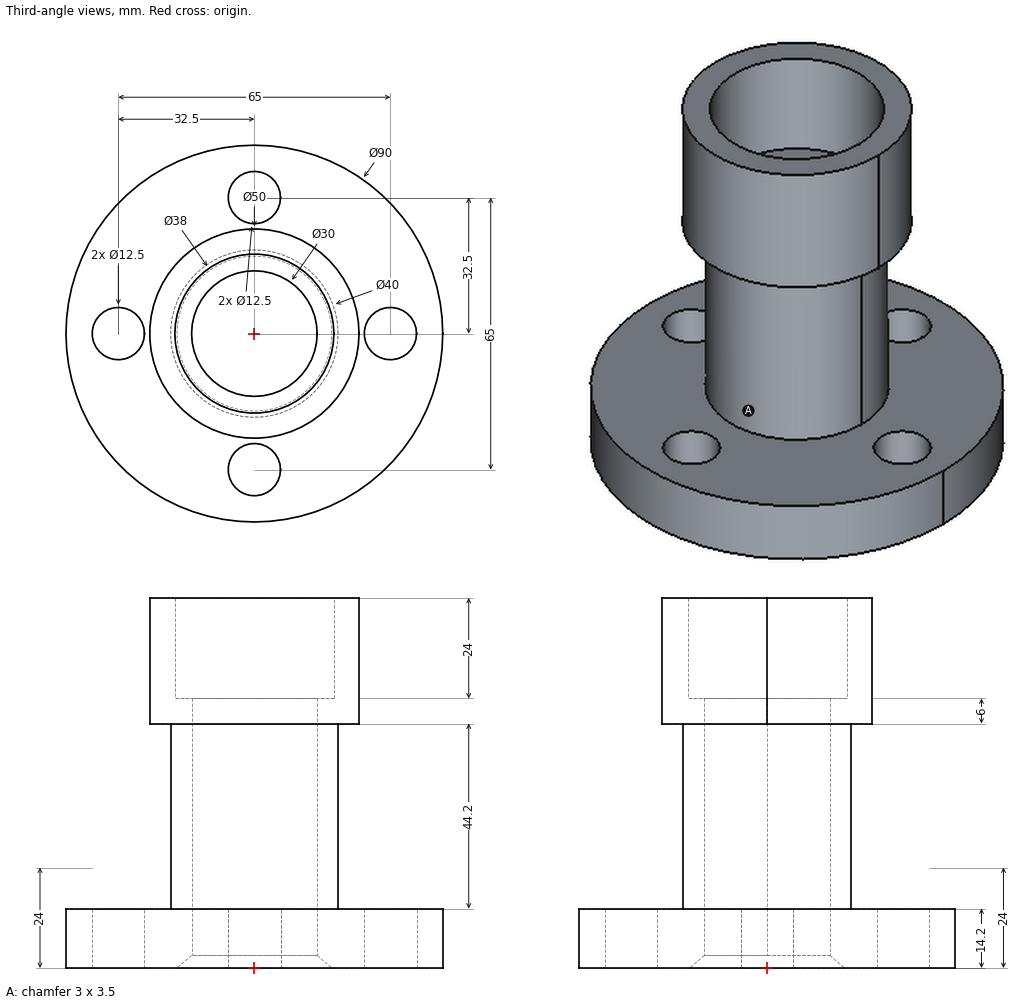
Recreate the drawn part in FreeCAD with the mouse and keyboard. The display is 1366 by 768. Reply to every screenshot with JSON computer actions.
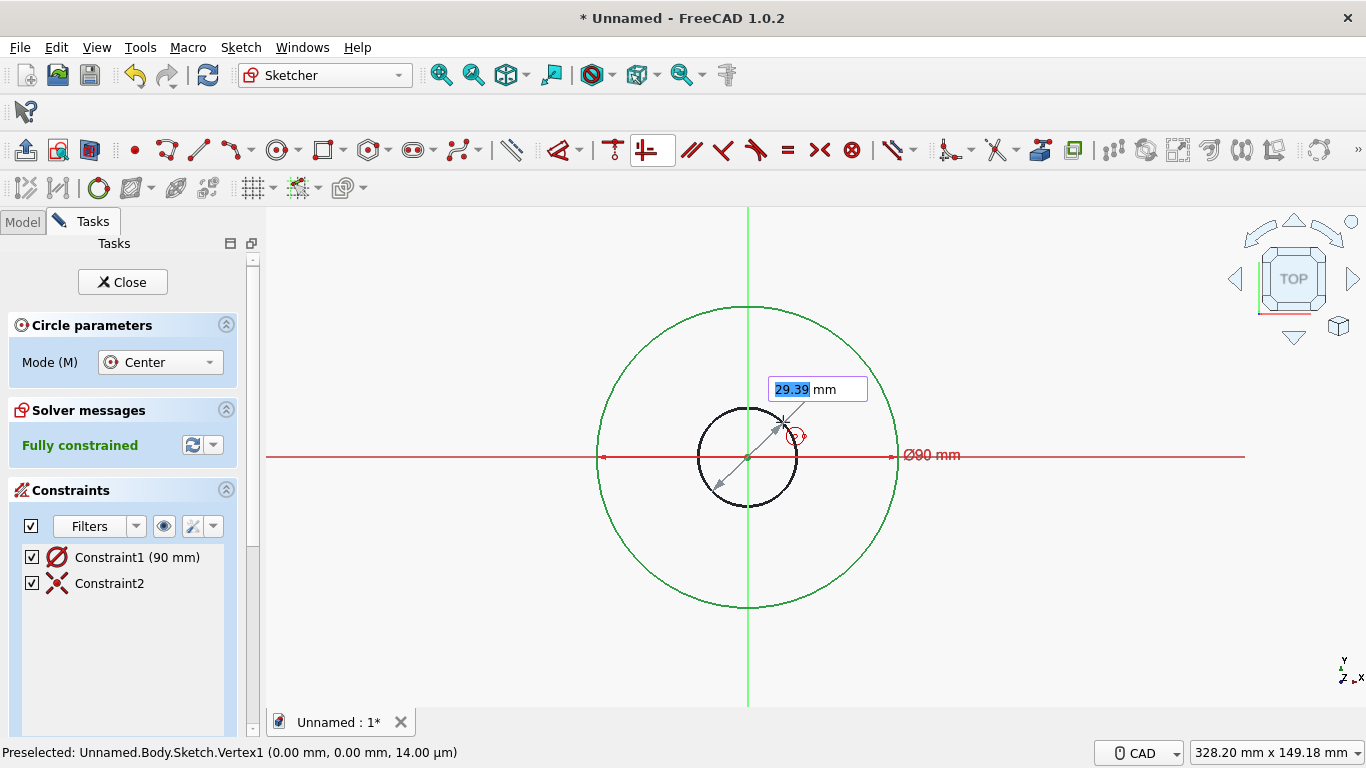
{"action": "type", "text": "30"}
{"action": "key", "text": "Return"}
{"action": "key", "text": "Escape"}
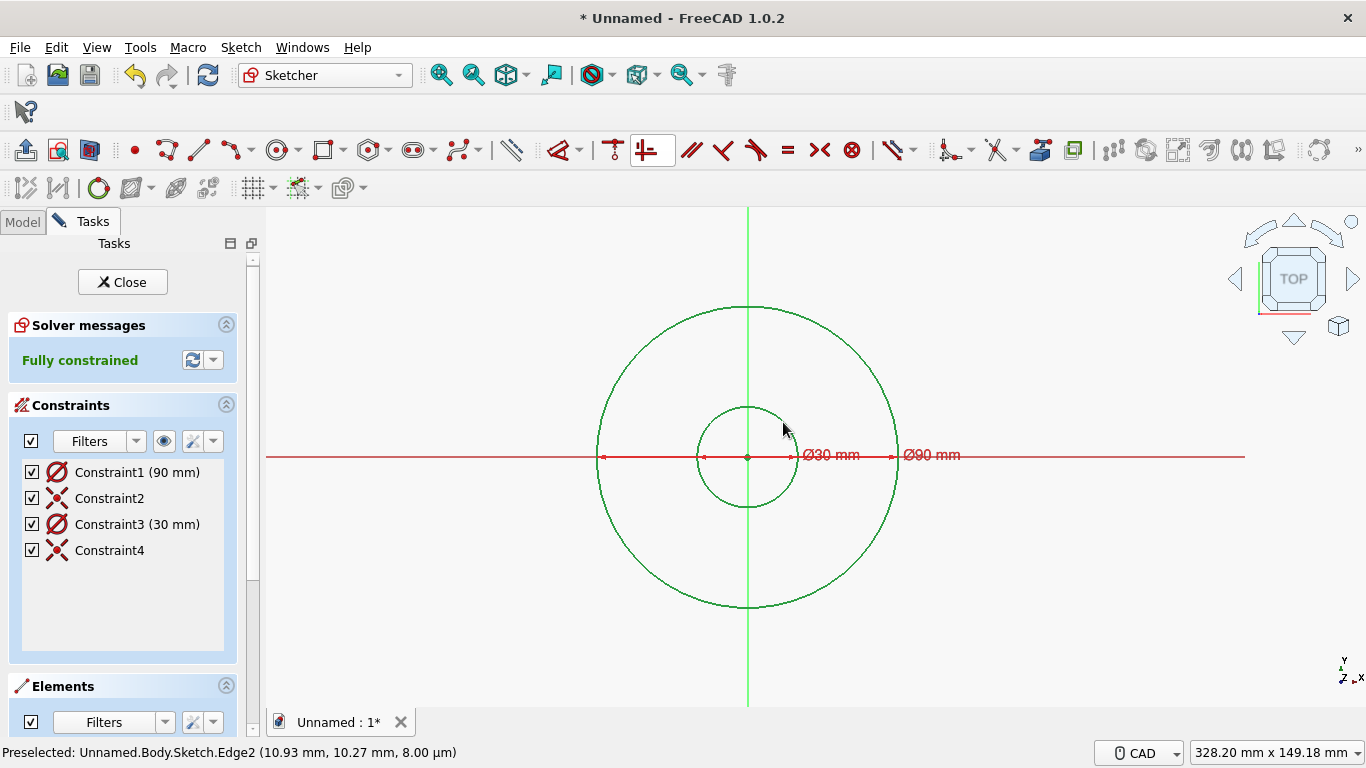
{"action": "left_click", "coordinate": [123, 282]}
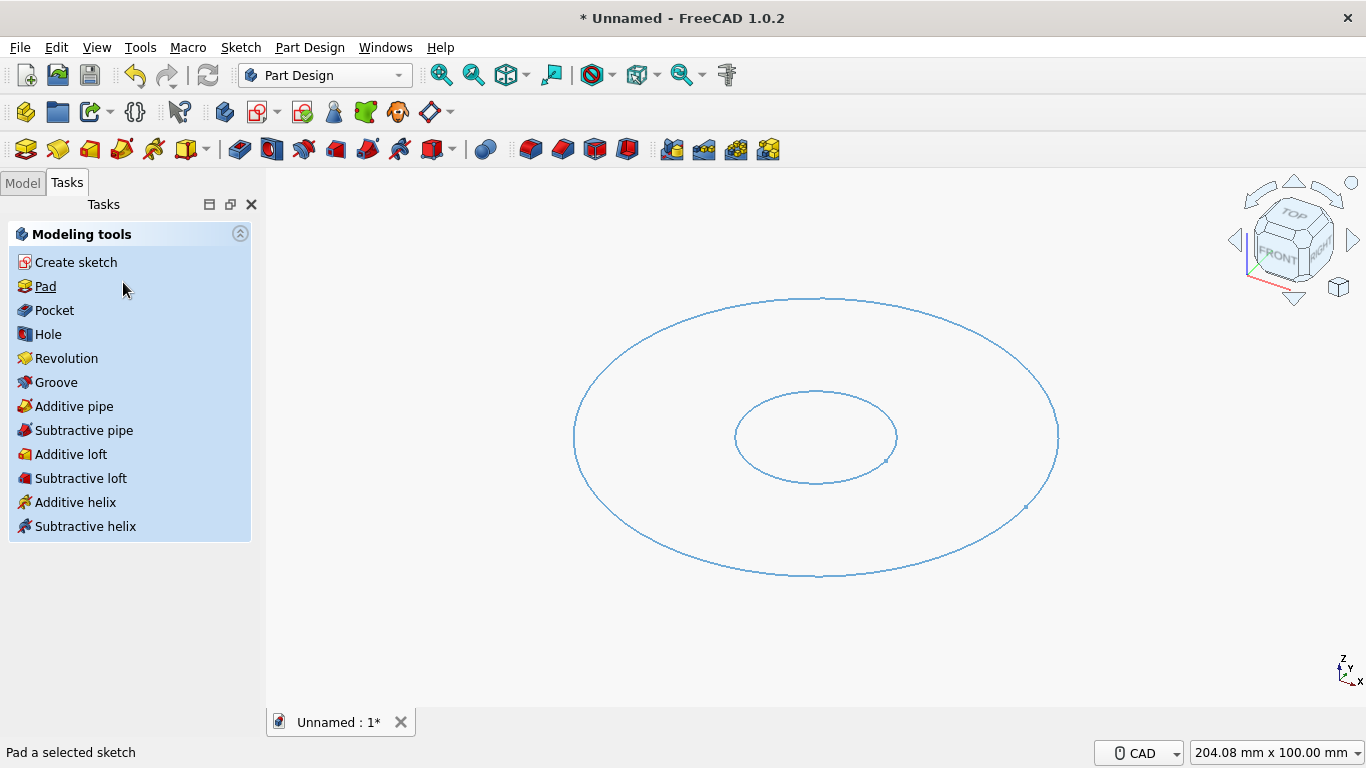
{"action": "left_click", "coordinate": [26, 150]}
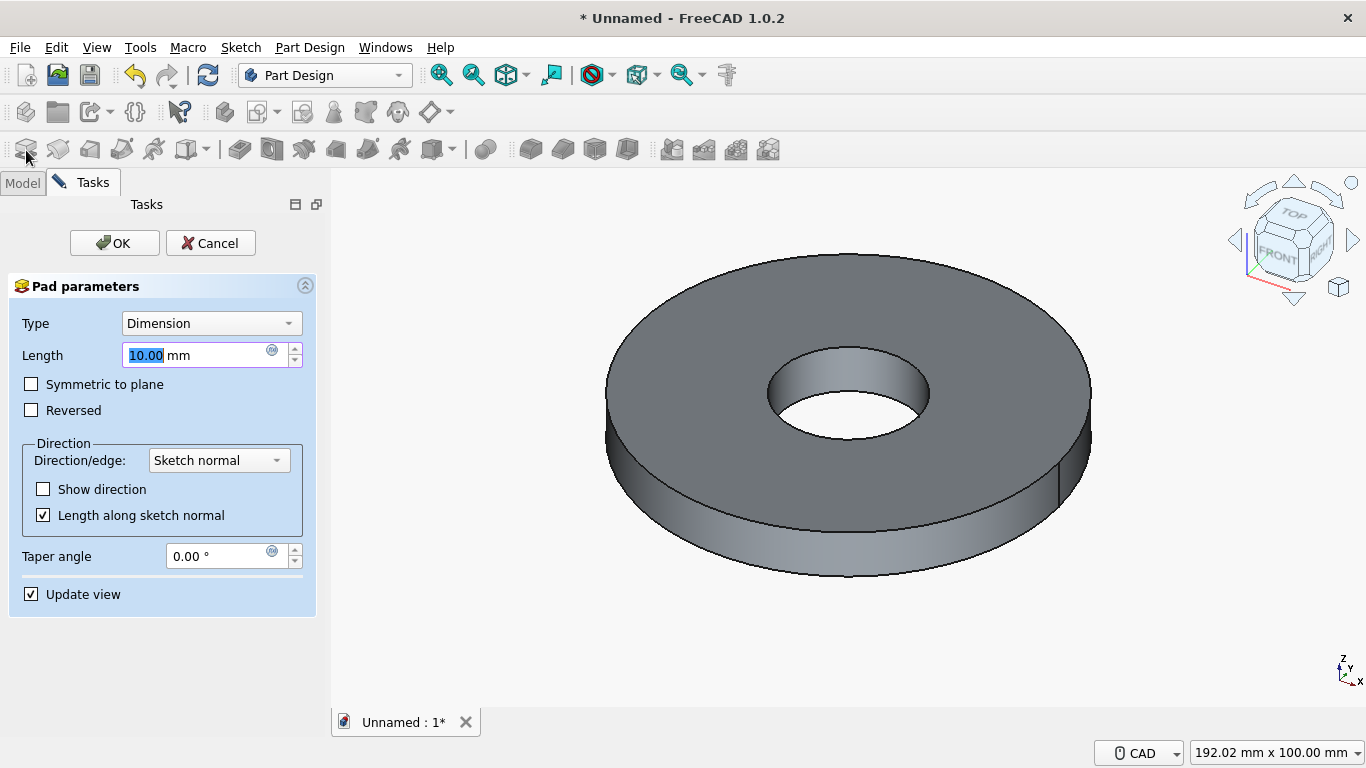
{"action": "type", "text": "14.2"}
{"action": "key", "text": "Tab"}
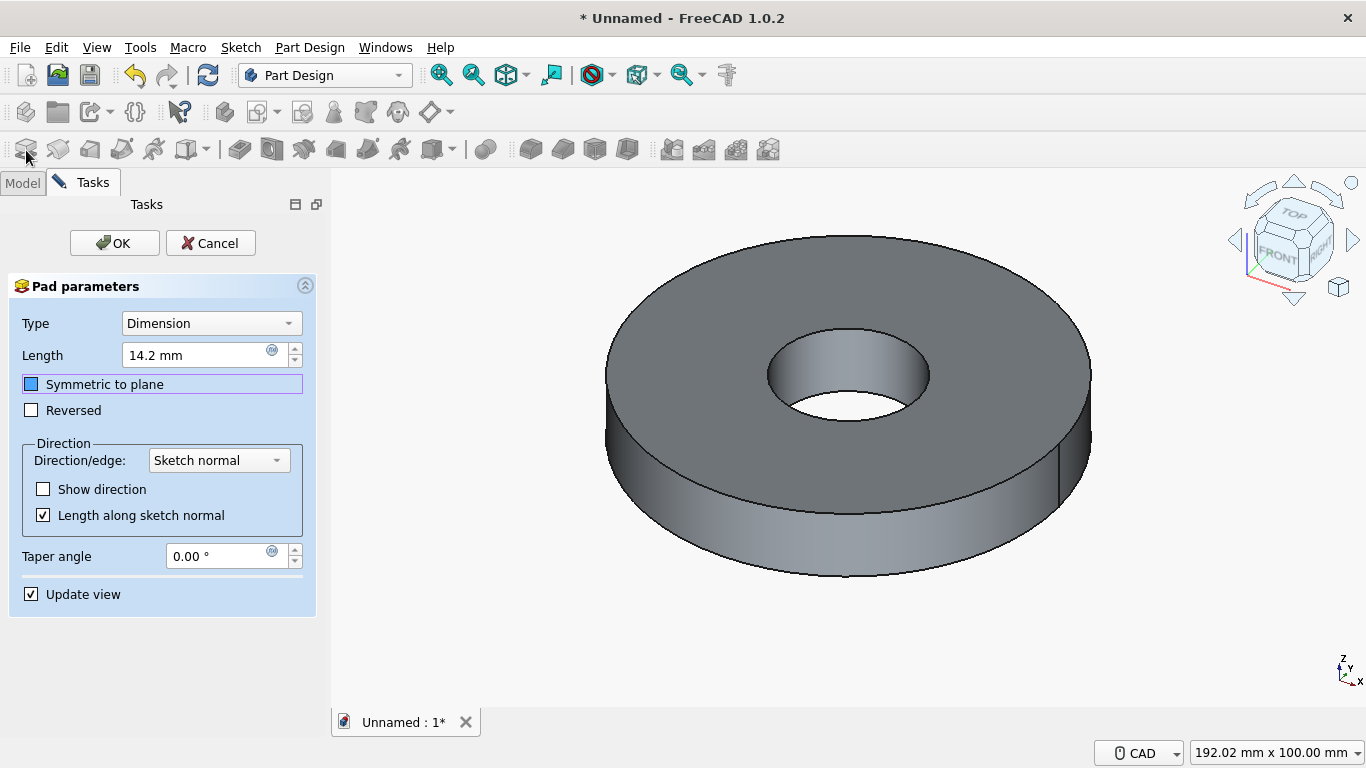
{"action": "left_click", "coordinate": [115, 243]}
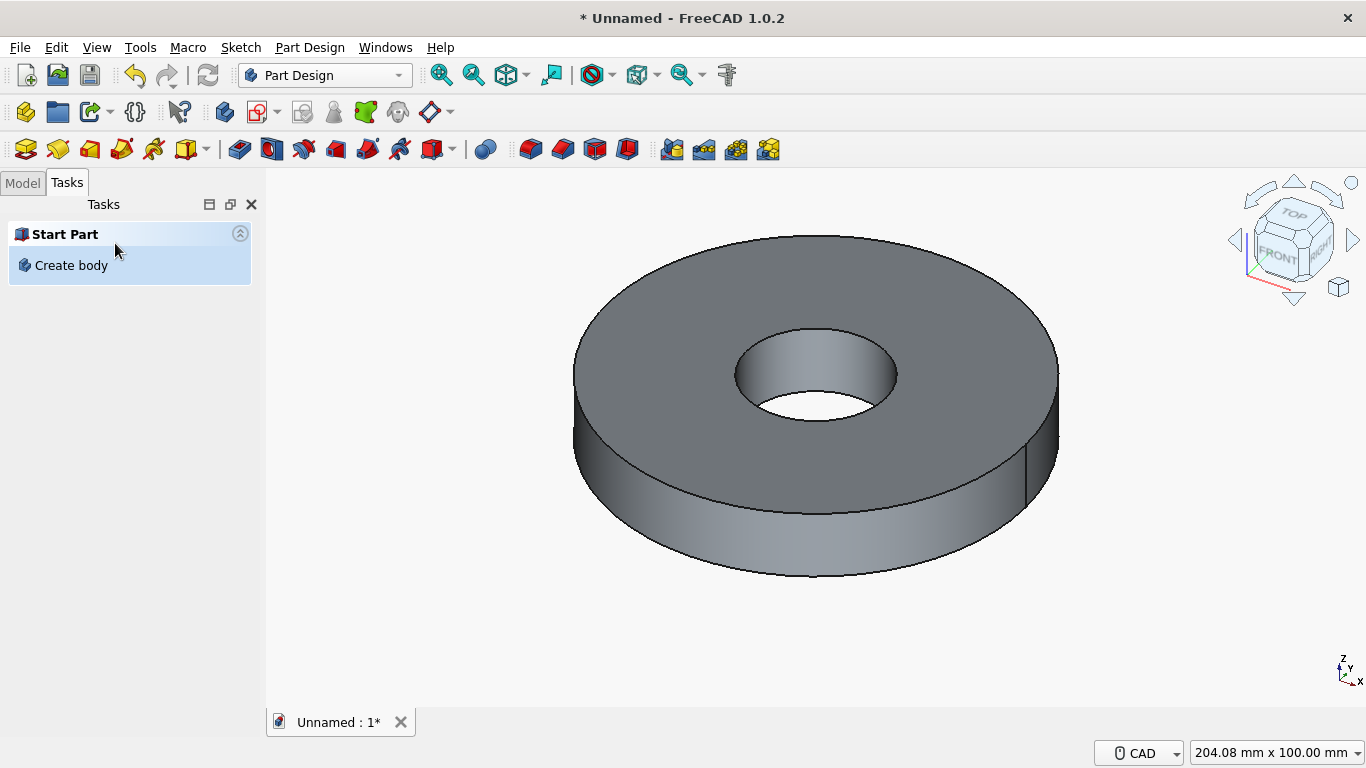
{"action": "left_click", "coordinate": [687, 423]}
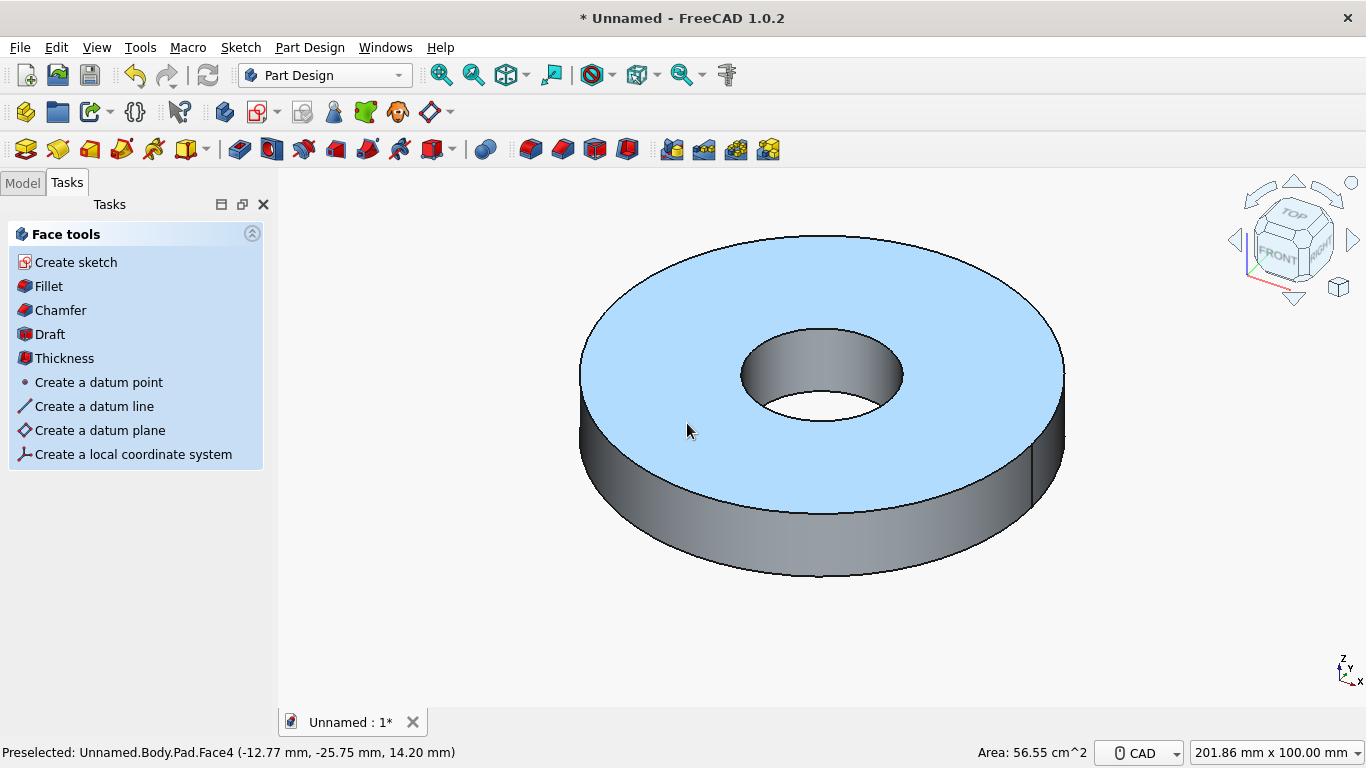
{"action": "left_click", "coordinate": [258, 112]}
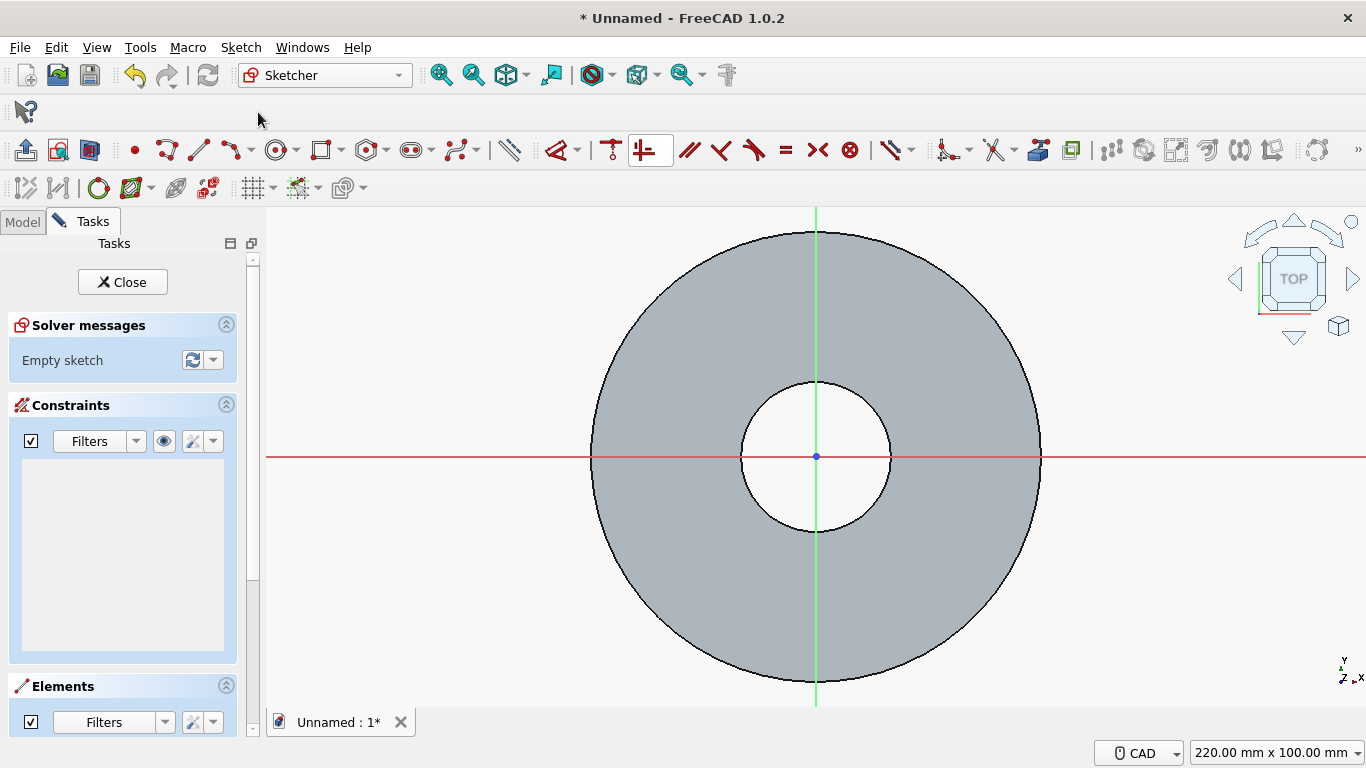
{"action": "scroll", "coordinate": [955, 457], "scroll_direction": "up", "scroll_amount": 2}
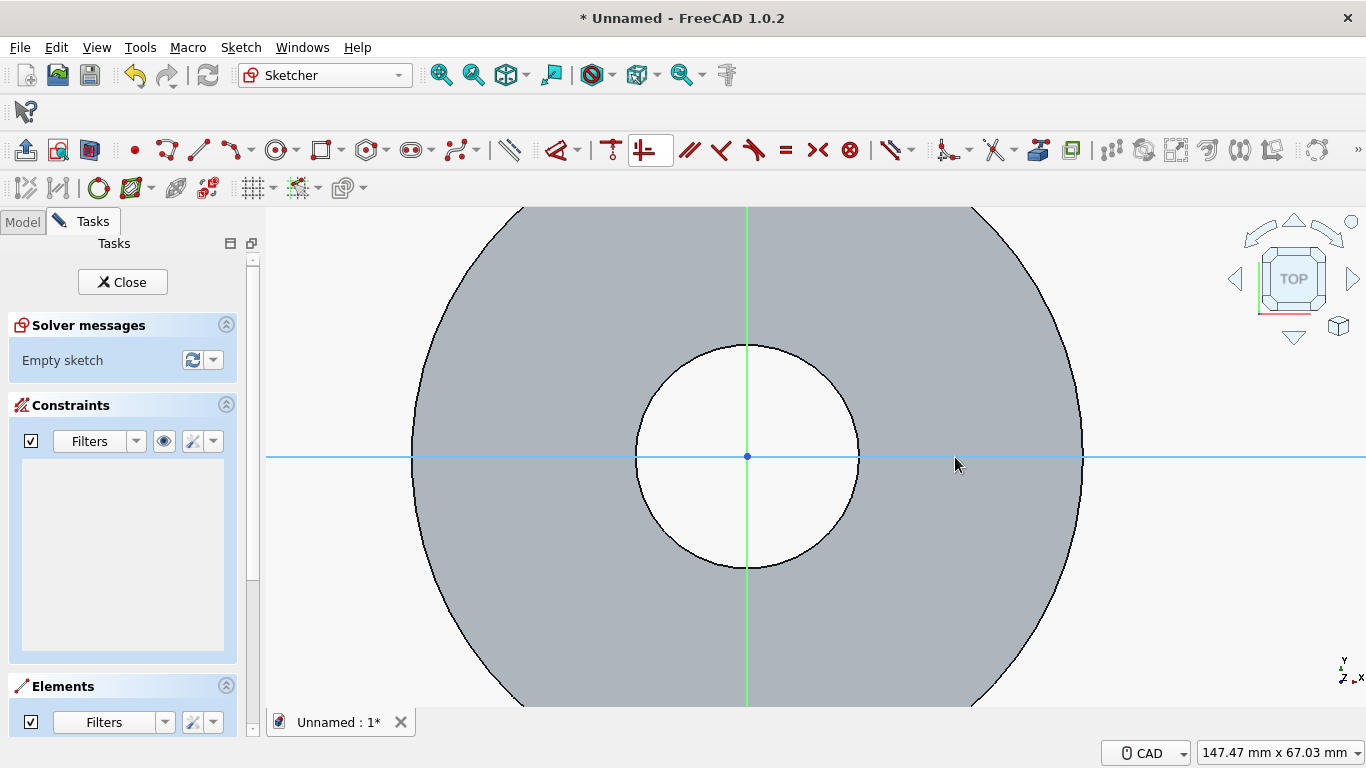
{"action": "left_click", "coordinate": [276, 150]}